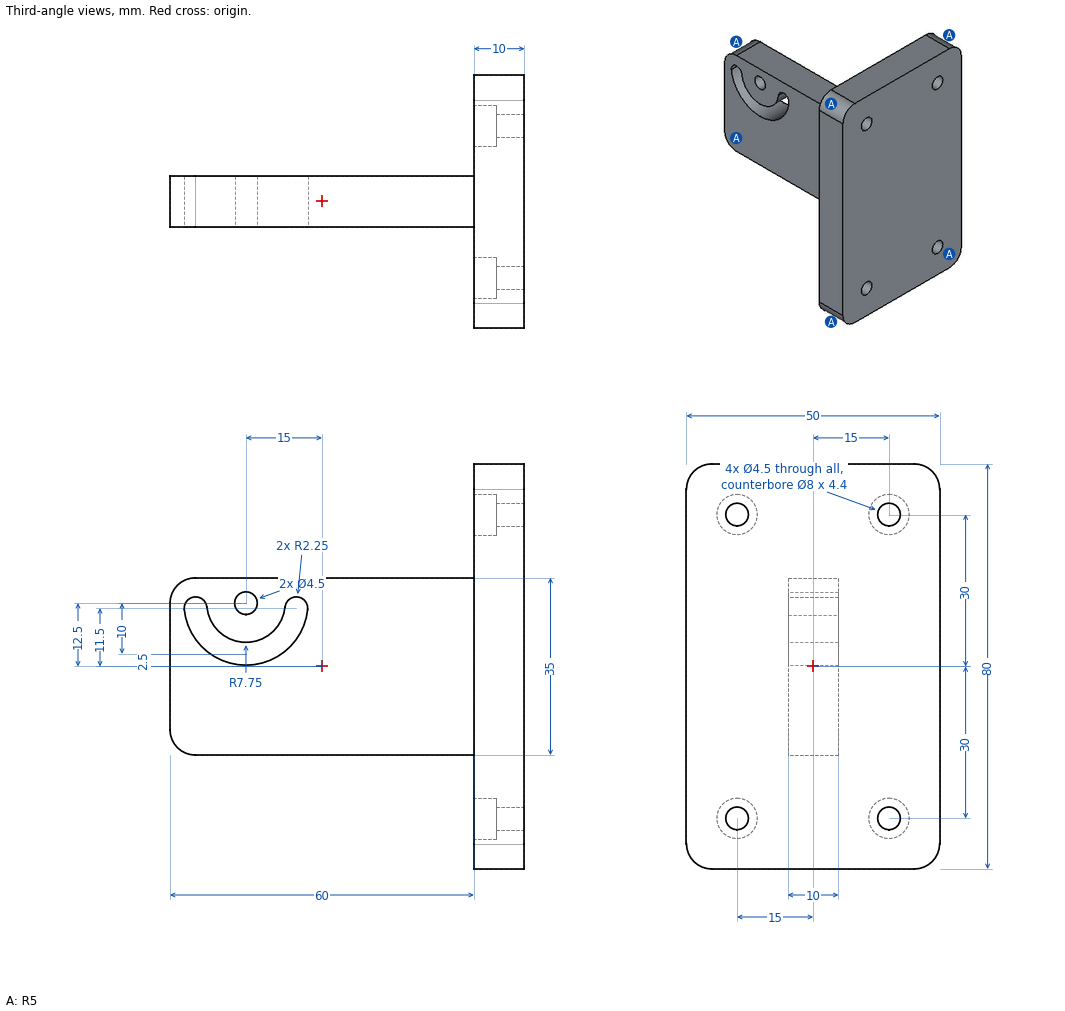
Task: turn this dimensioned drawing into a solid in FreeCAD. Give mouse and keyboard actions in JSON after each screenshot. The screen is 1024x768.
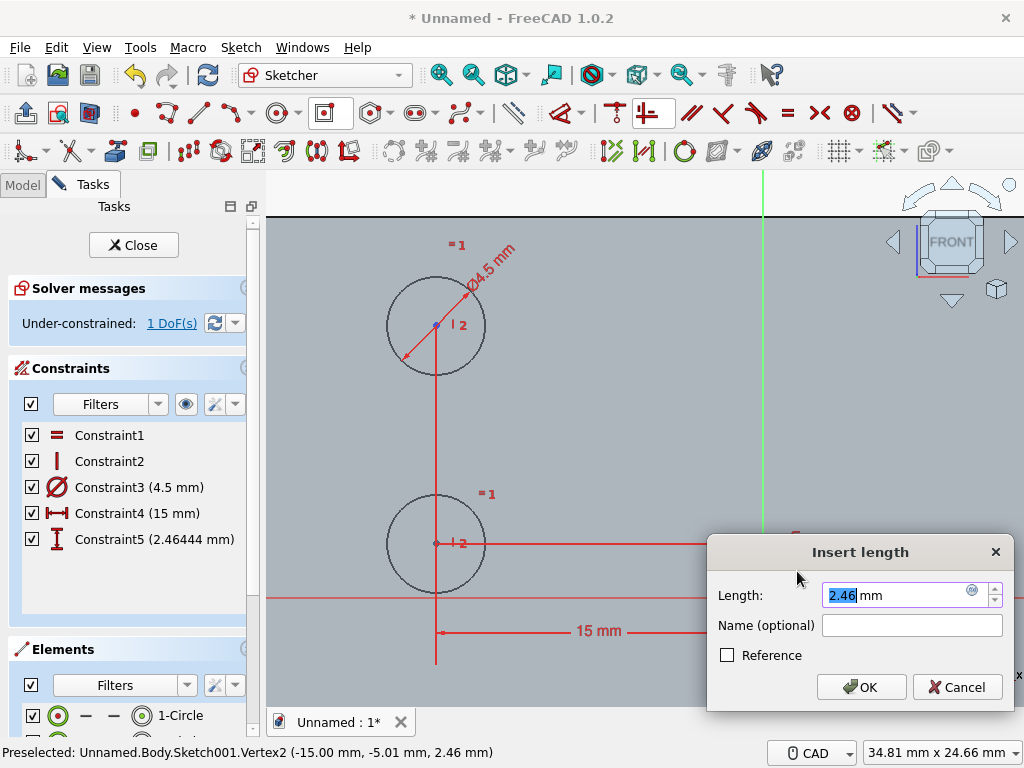
{"action": "type", "text": "2.5"}
{"action": "key", "text": "Return"}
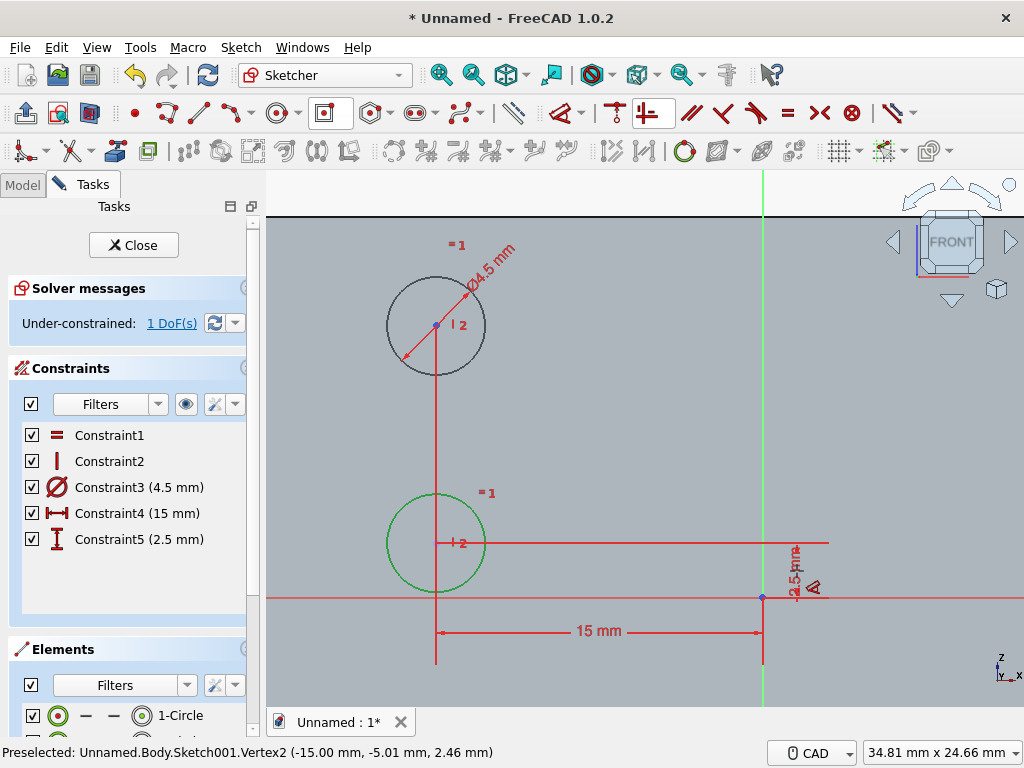
{"action": "left_click", "coordinate": [436, 326]}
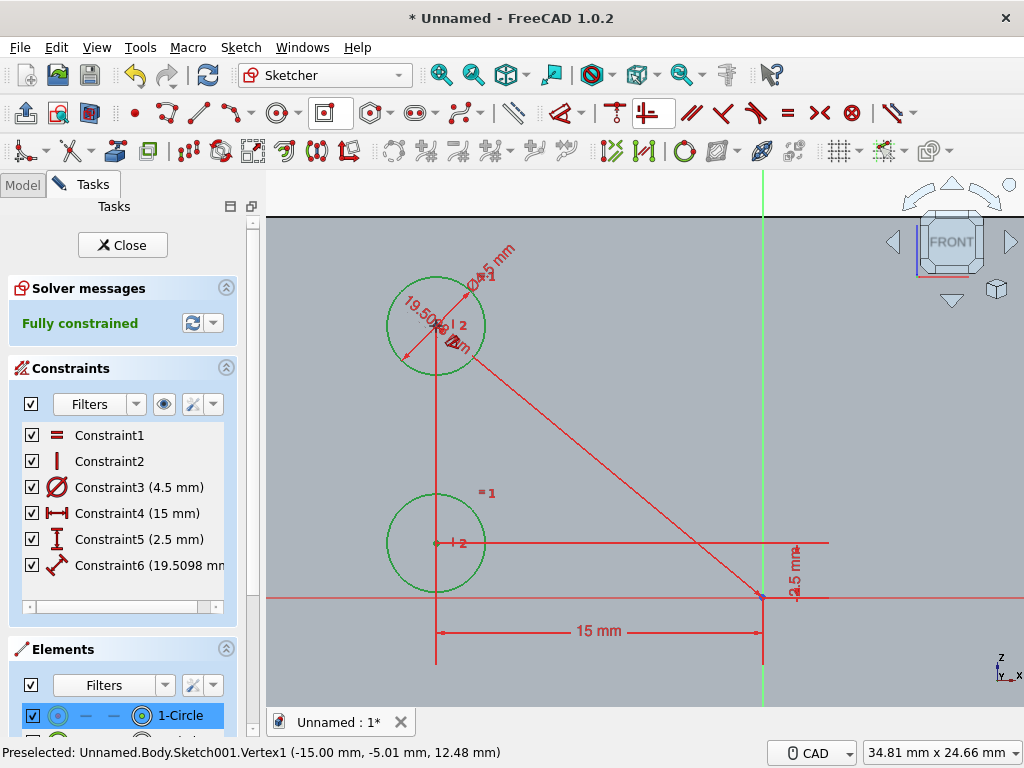
{"action": "left_click", "coordinate": [436, 543]}
{"action": "left_click", "coordinate": [402, 435]}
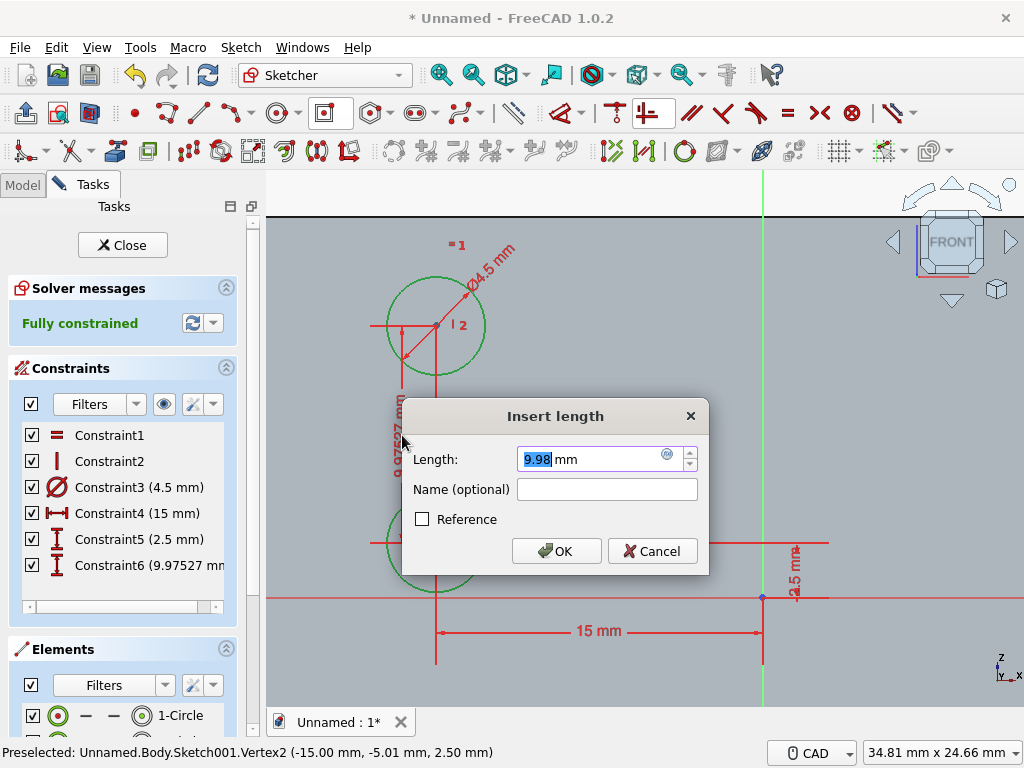
{"action": "type", "text": "10"}
{"action": "key", "text": "Return"}
{"action": "key", "text": "Escape"}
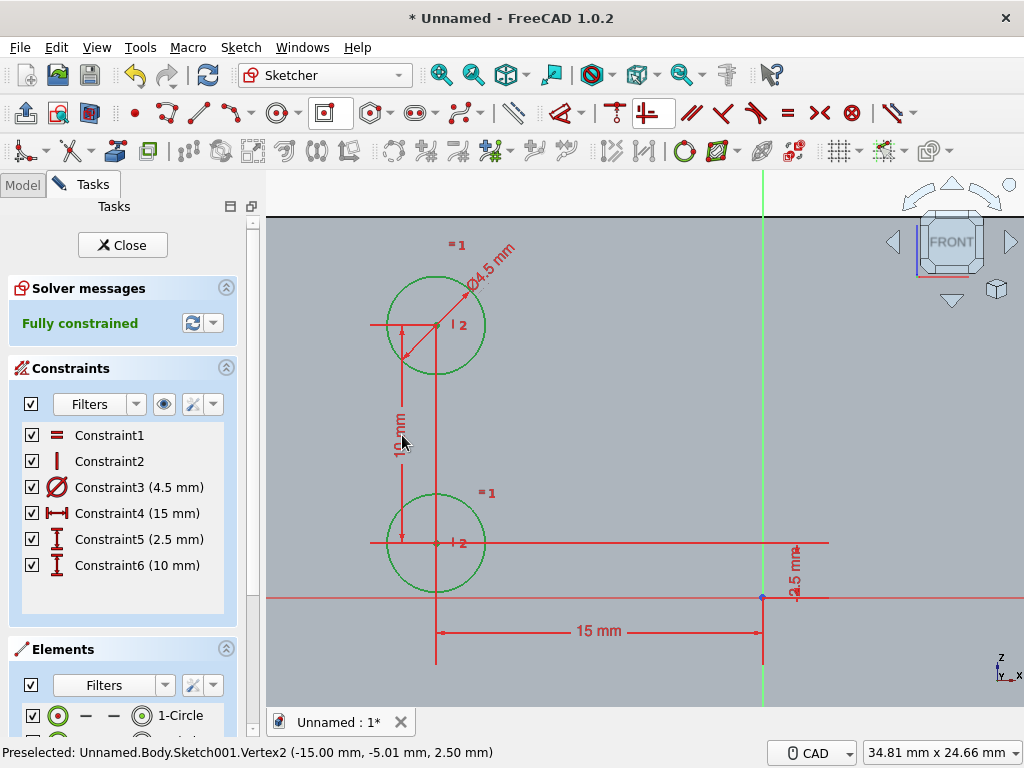
{"action": "left_click", "coordinate": [123, 245]}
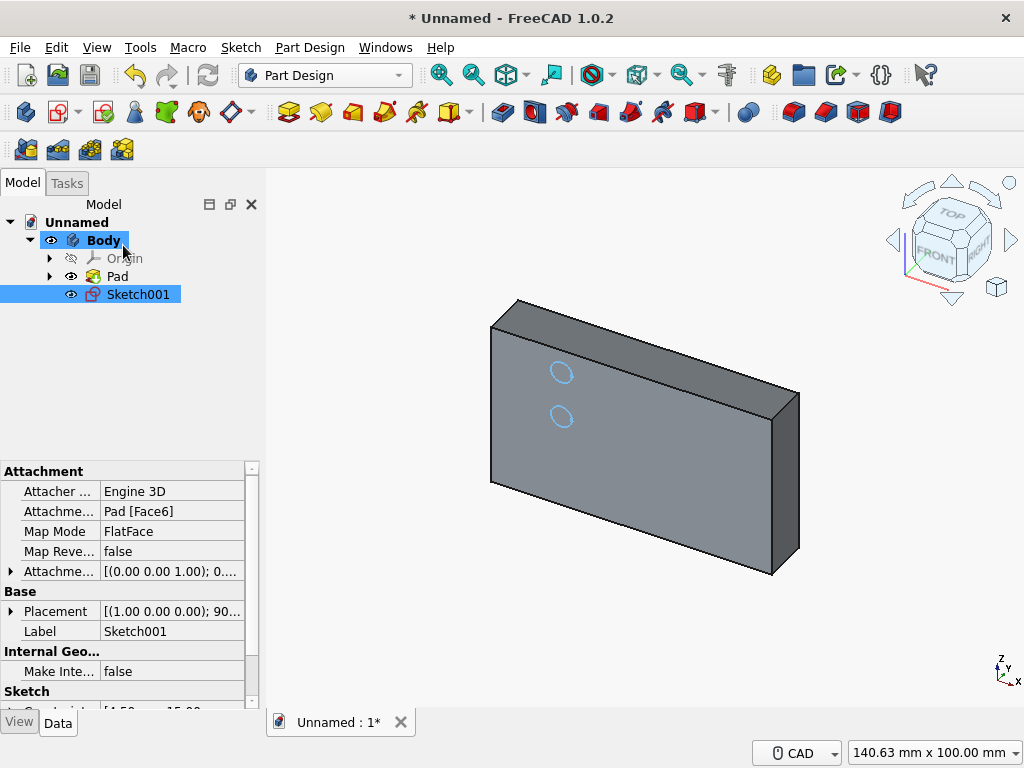
{"action": "left_click", "coordinate": [504, 112]}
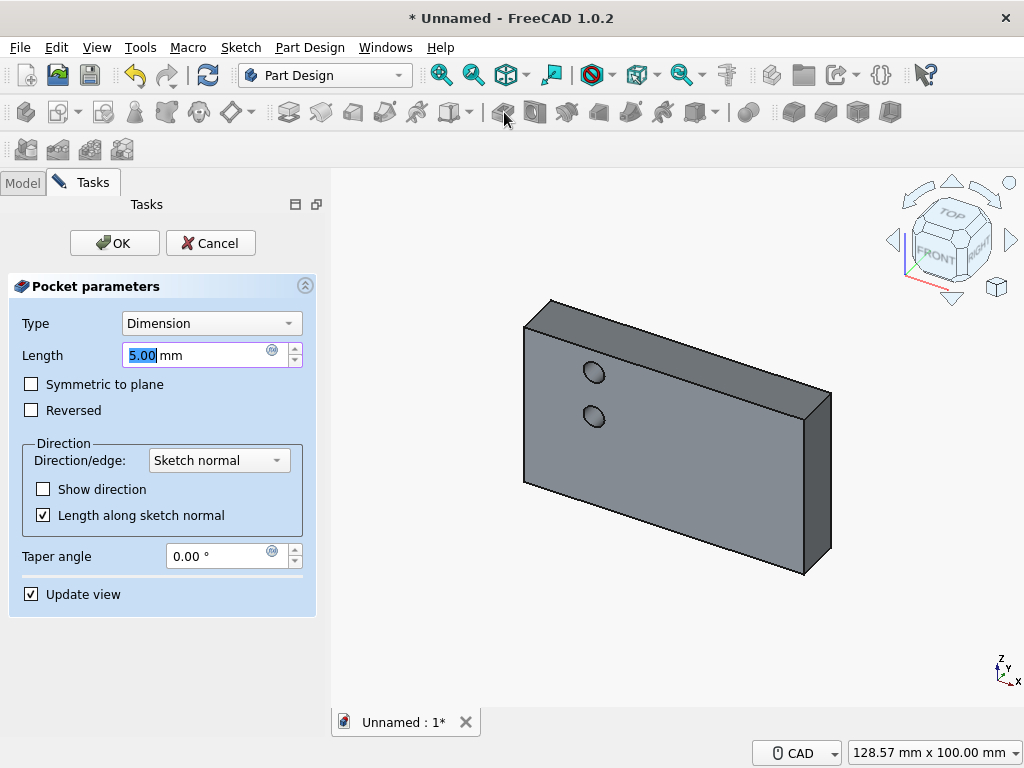
{"action": "left_click", "coordinate": [212, 324]}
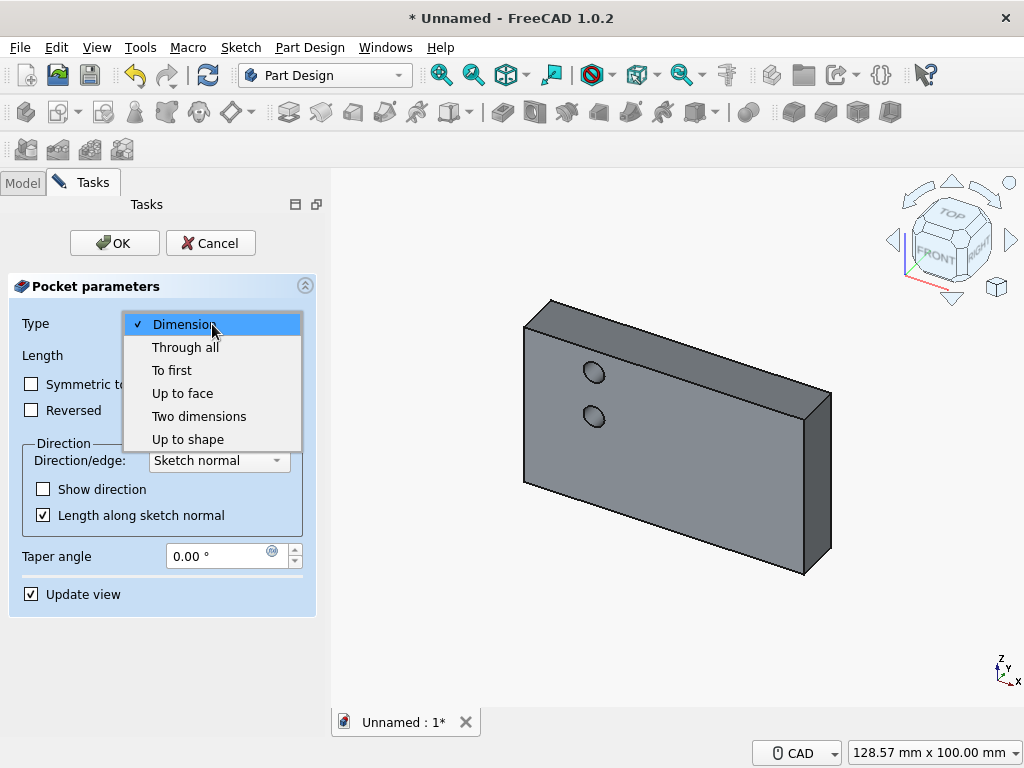
{"action": "left_click", "coordinate": [212, 348]}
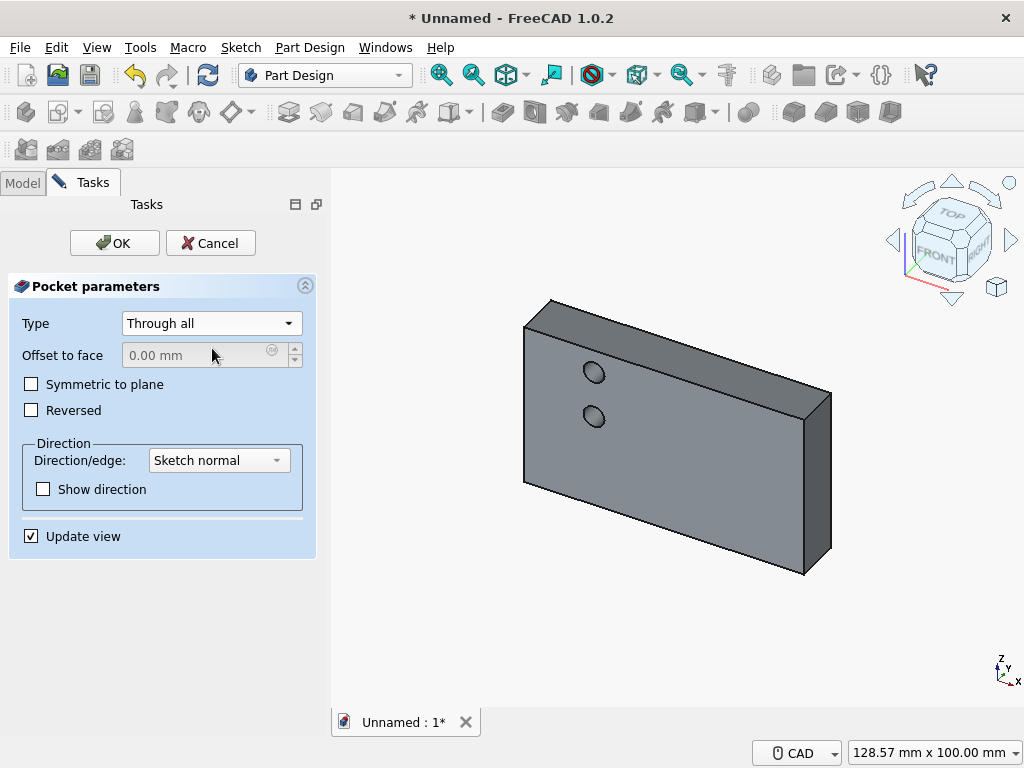
{"action": "left_click", "coordinate": [115, 243]}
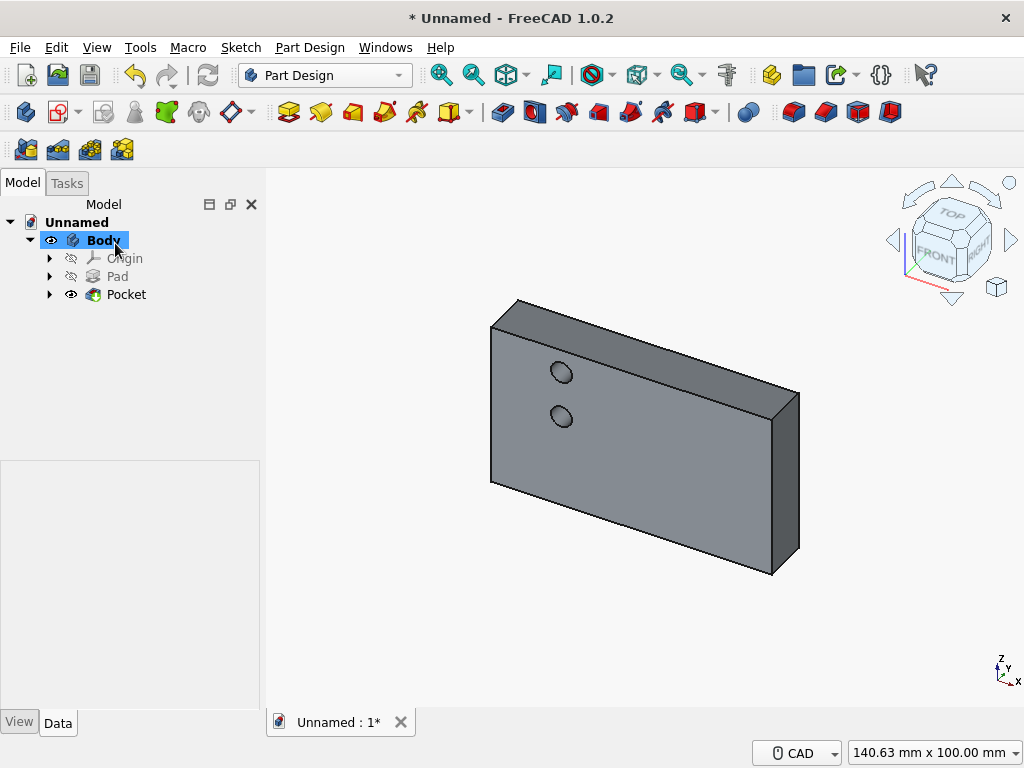
{"action": "left_click", "coordinate": [672, 463]}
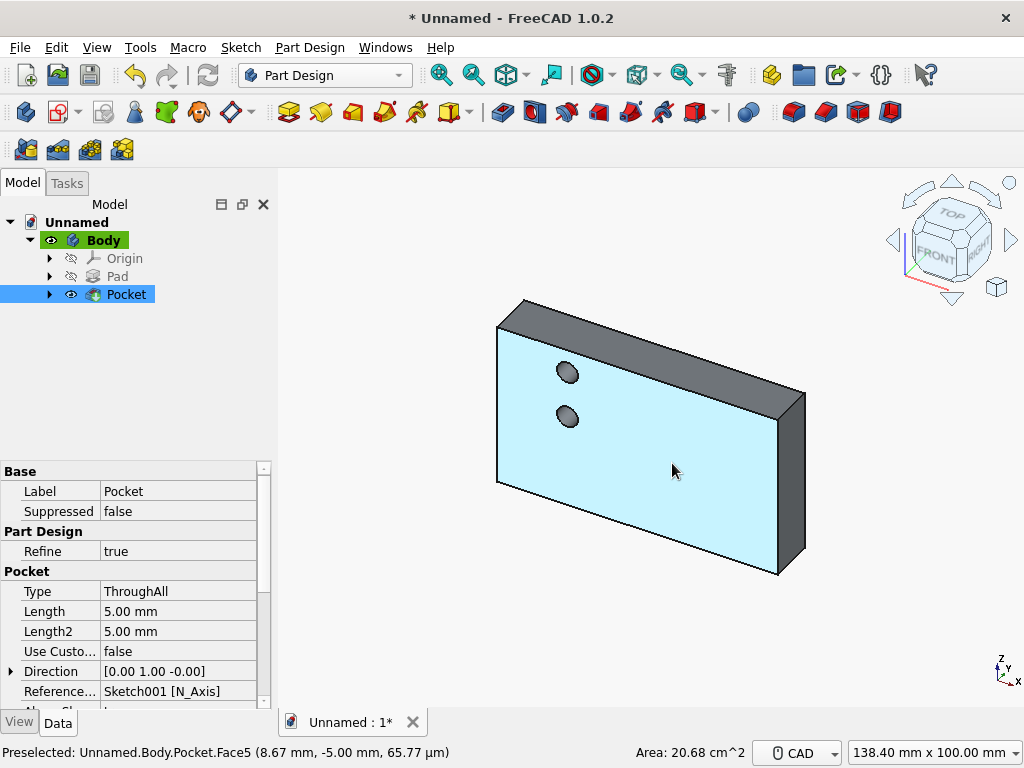
{"action": "left_click", "coordinate": [58, 112]}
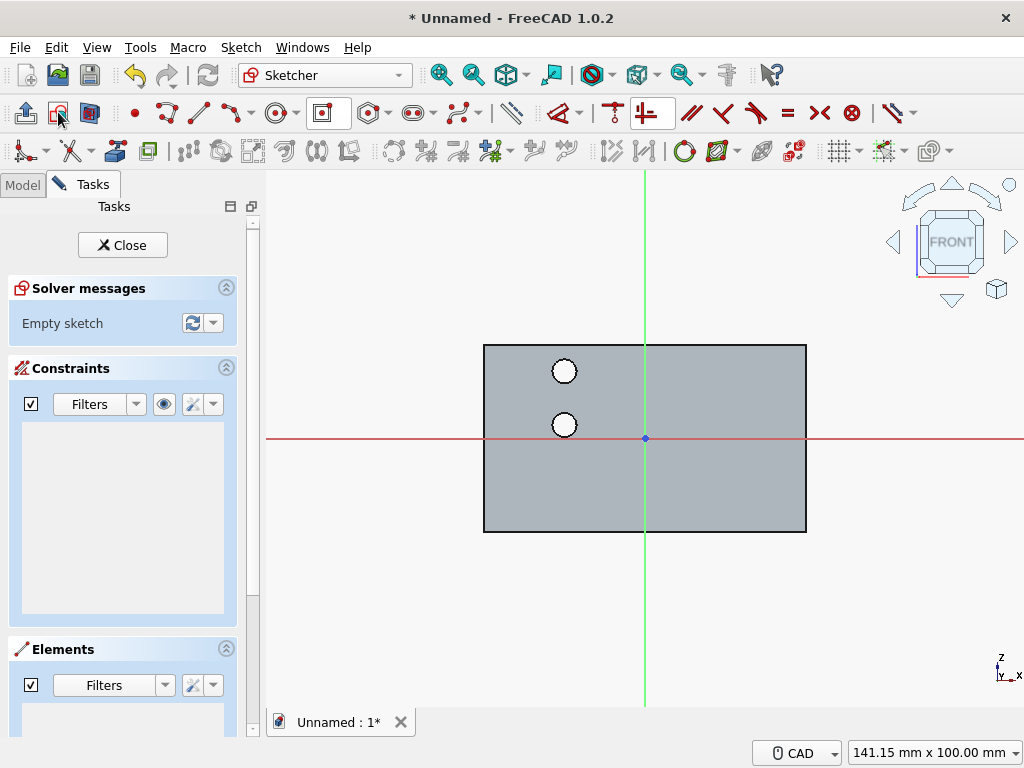
{"action": "scroll", "coordinate": [569, 380], "scroll_direction": "up", "scroll_amount": 5}